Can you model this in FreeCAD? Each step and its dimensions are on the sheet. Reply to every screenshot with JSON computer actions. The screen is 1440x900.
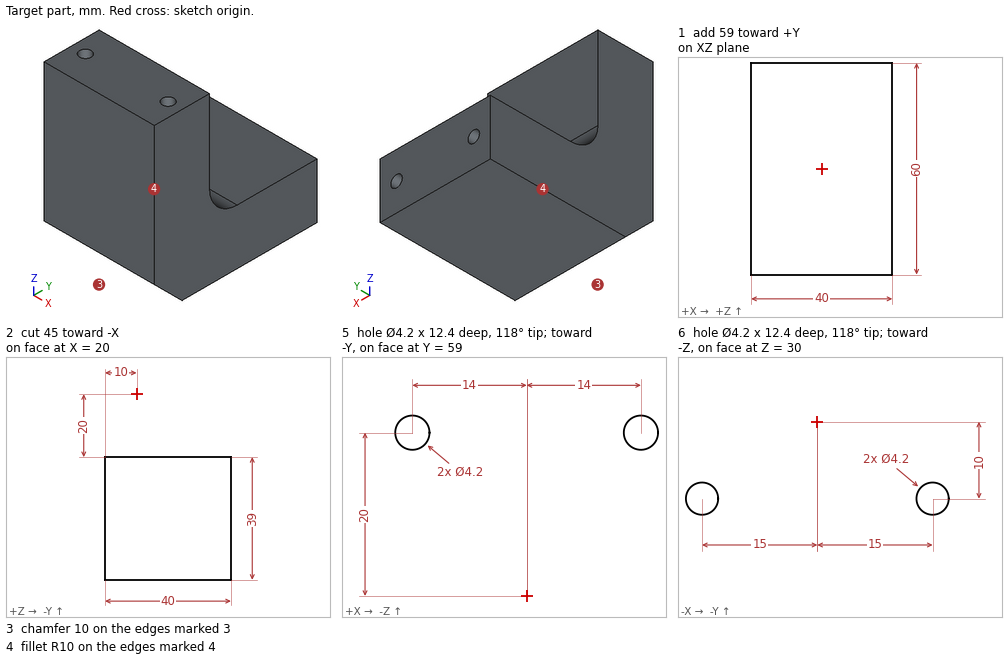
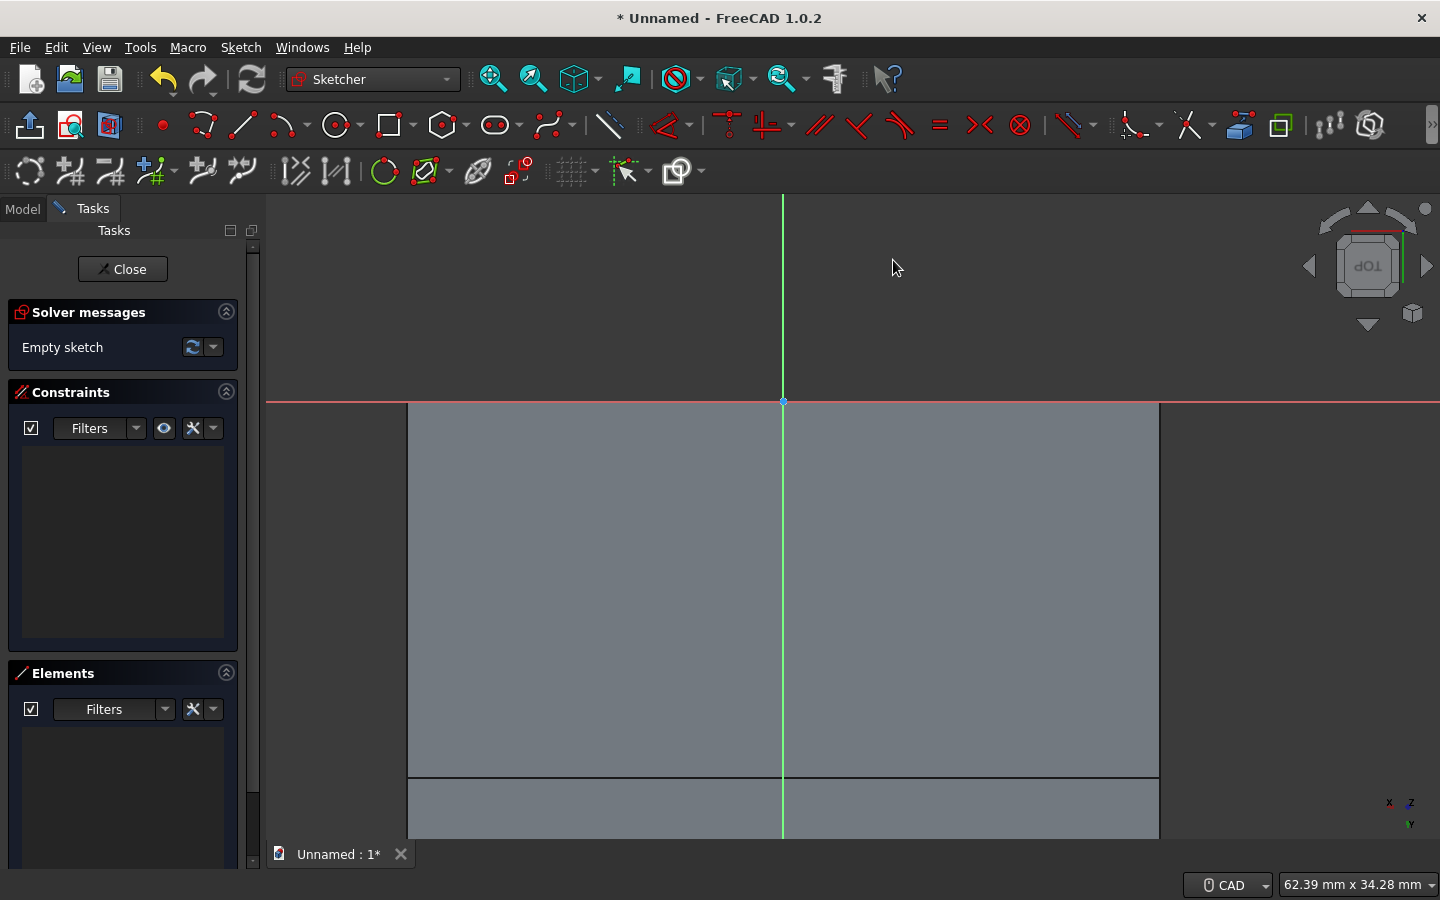
{"action": "left_click", "coordinate": [336, 126]}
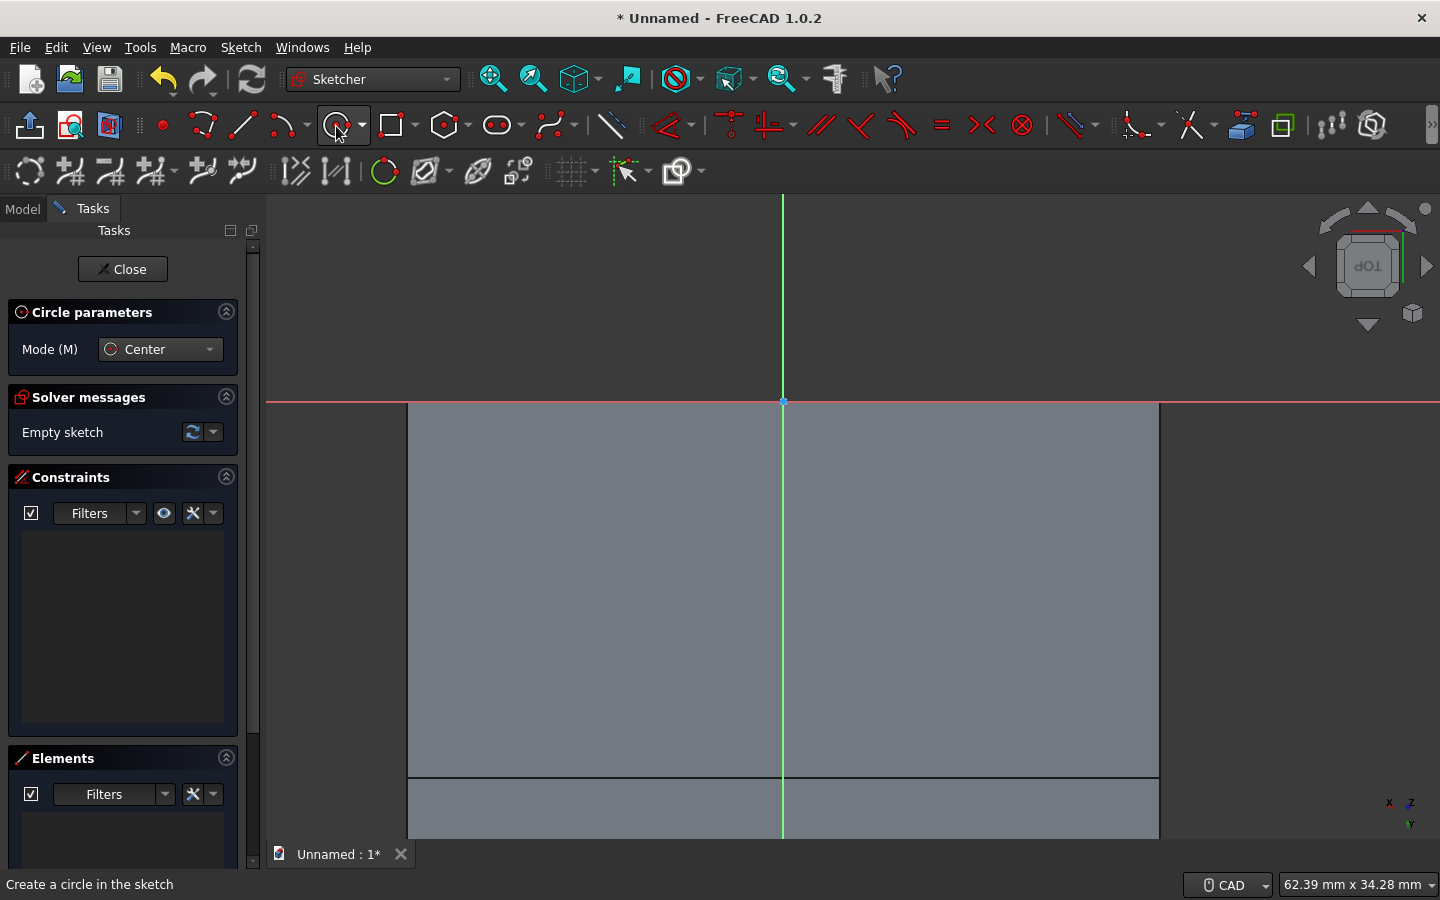
{"action": "left_click", "coordinate": [1066, 590]}
{"action": "mouse_move", "coordinate": [1094, 562]}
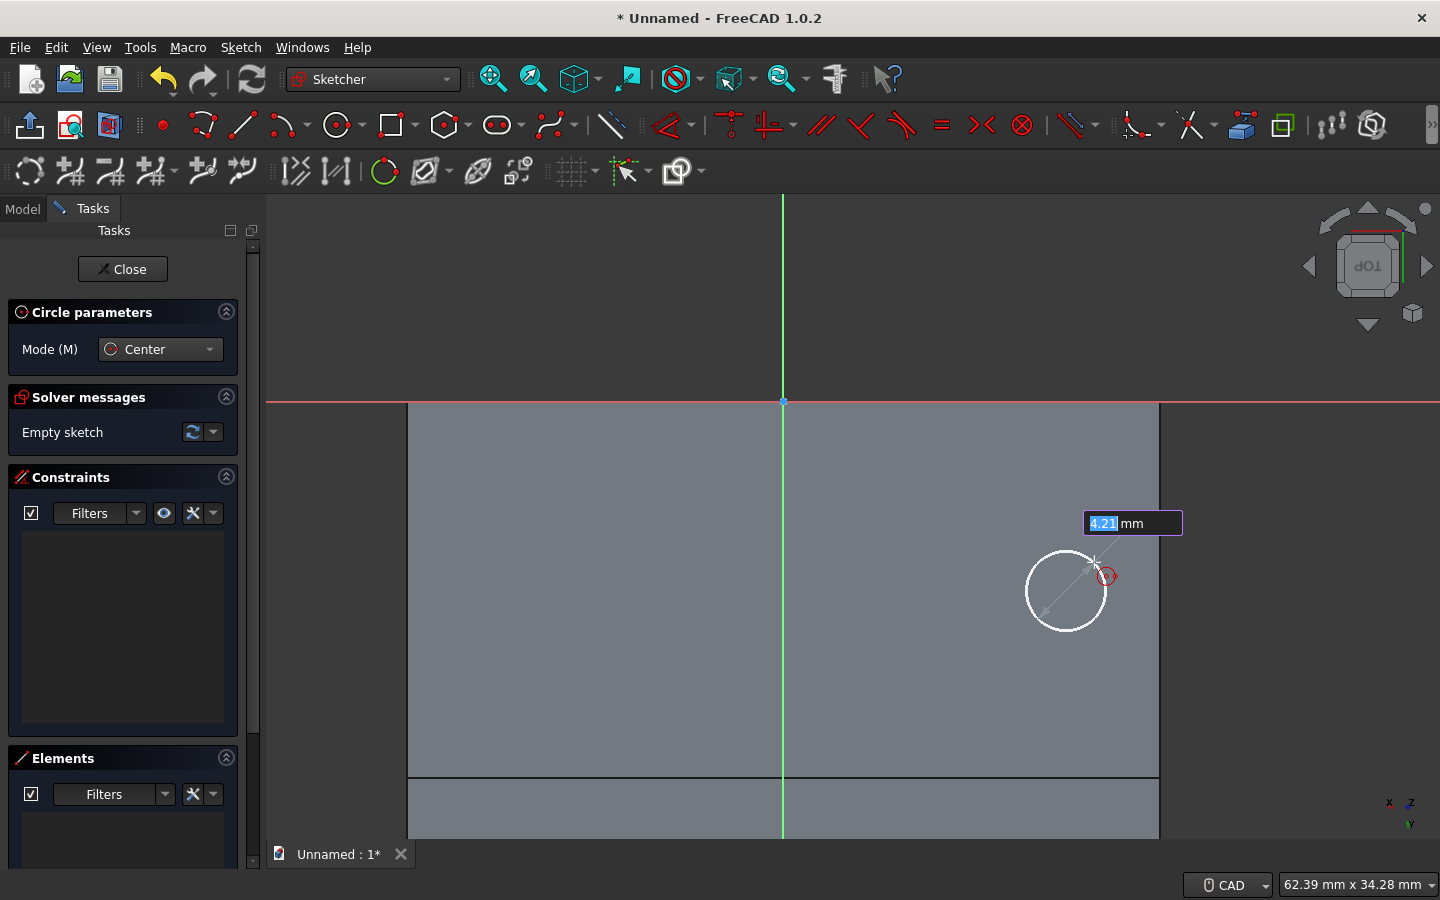
{"action": "type", "text": "4.2"}
{"action": "key", "text": "Return"}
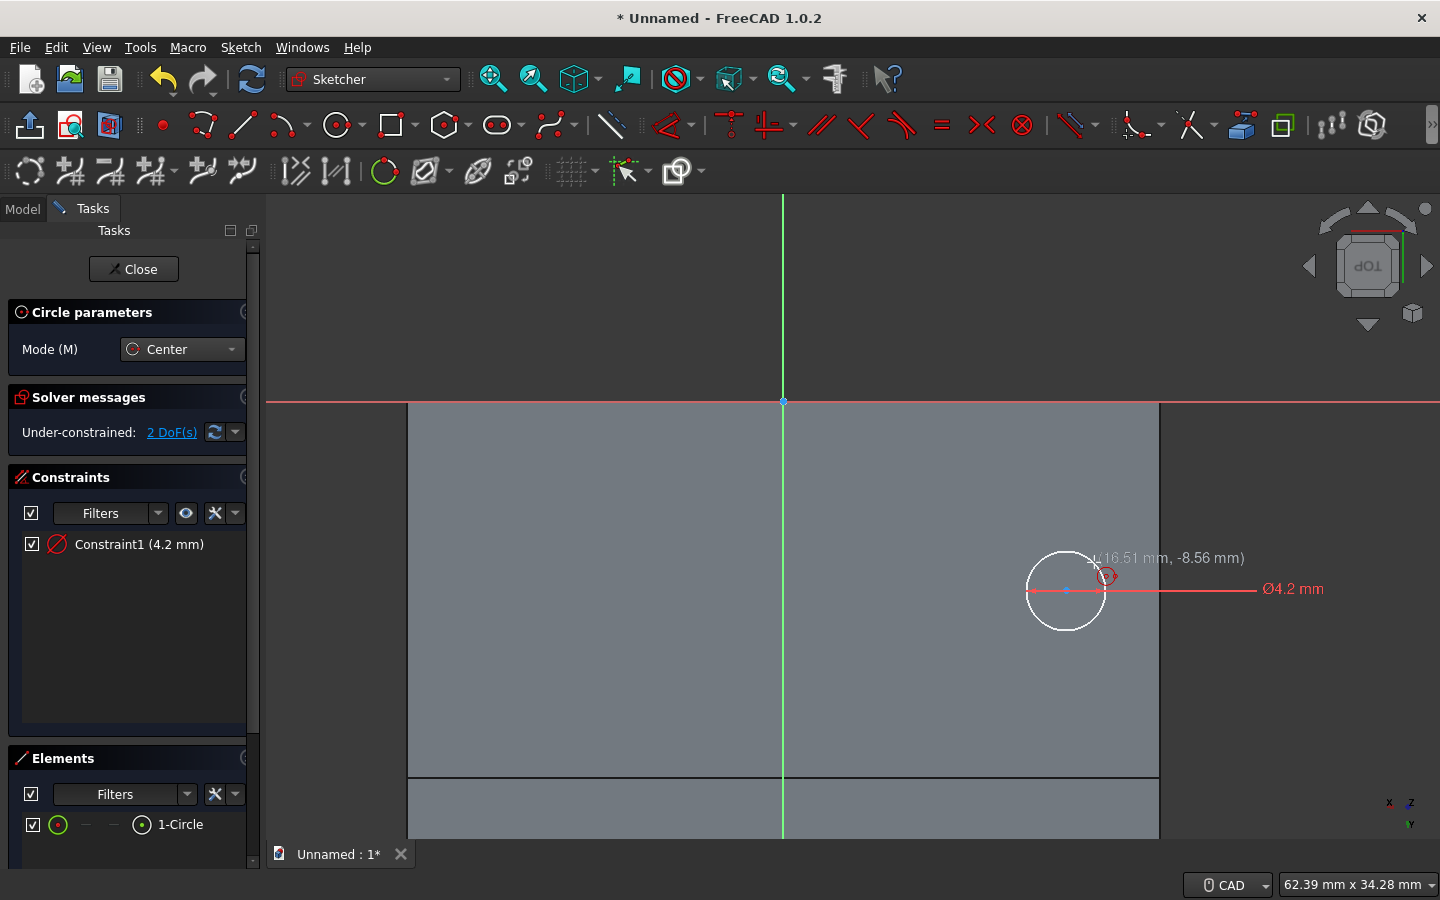
{"action": "left_click", "coordinate": [501, 590]}
{"action": "mouse_move", "coordinate": [529, 562]}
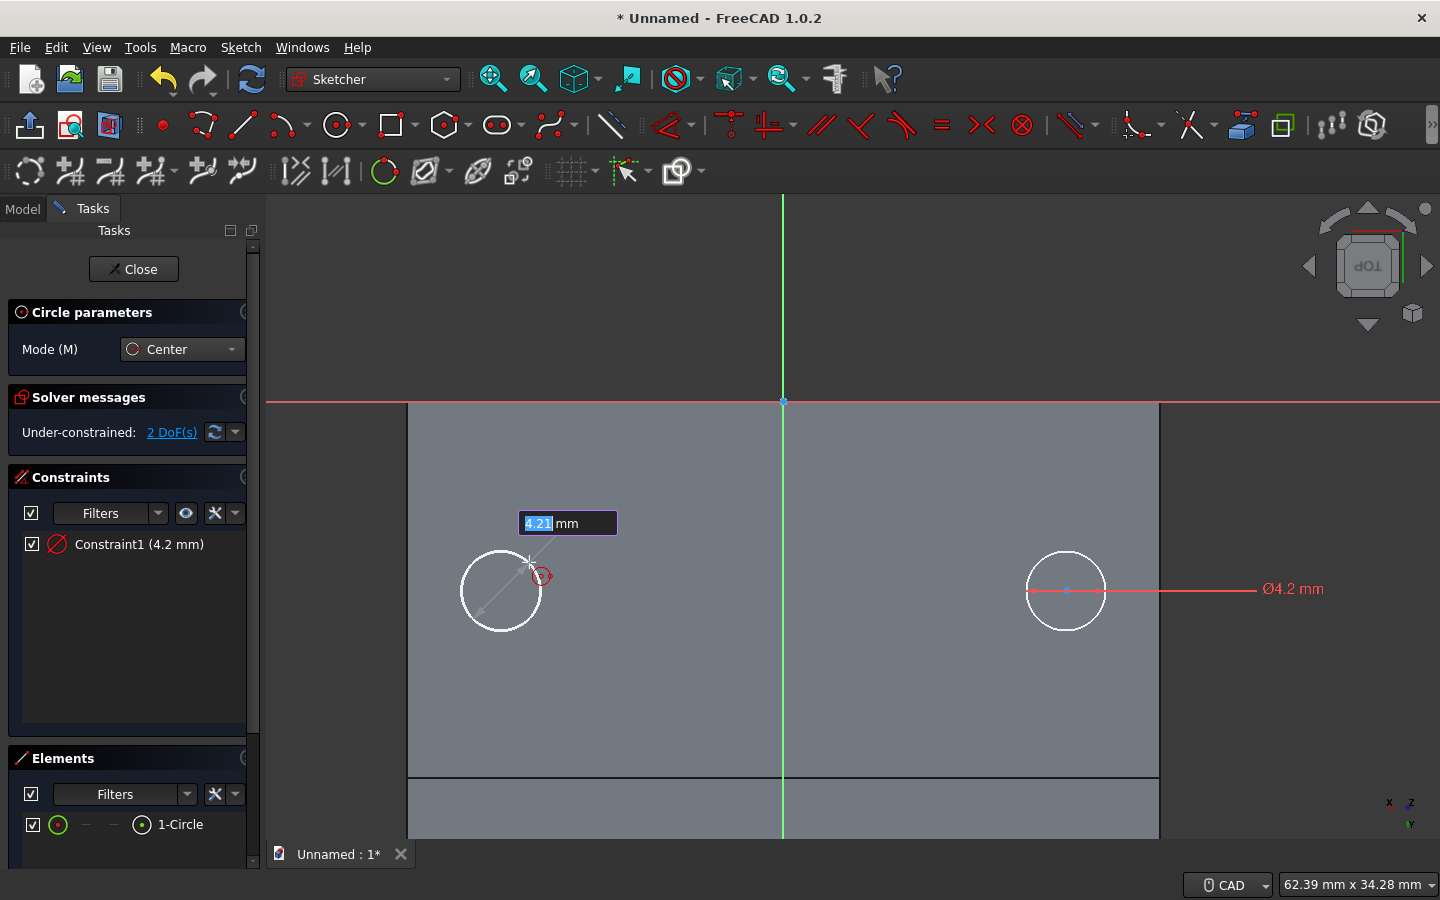
{"action": "type", "text": "4.2"}
{"action": "key", "text": "Return"}
{"action": "key", "text": "Escape"}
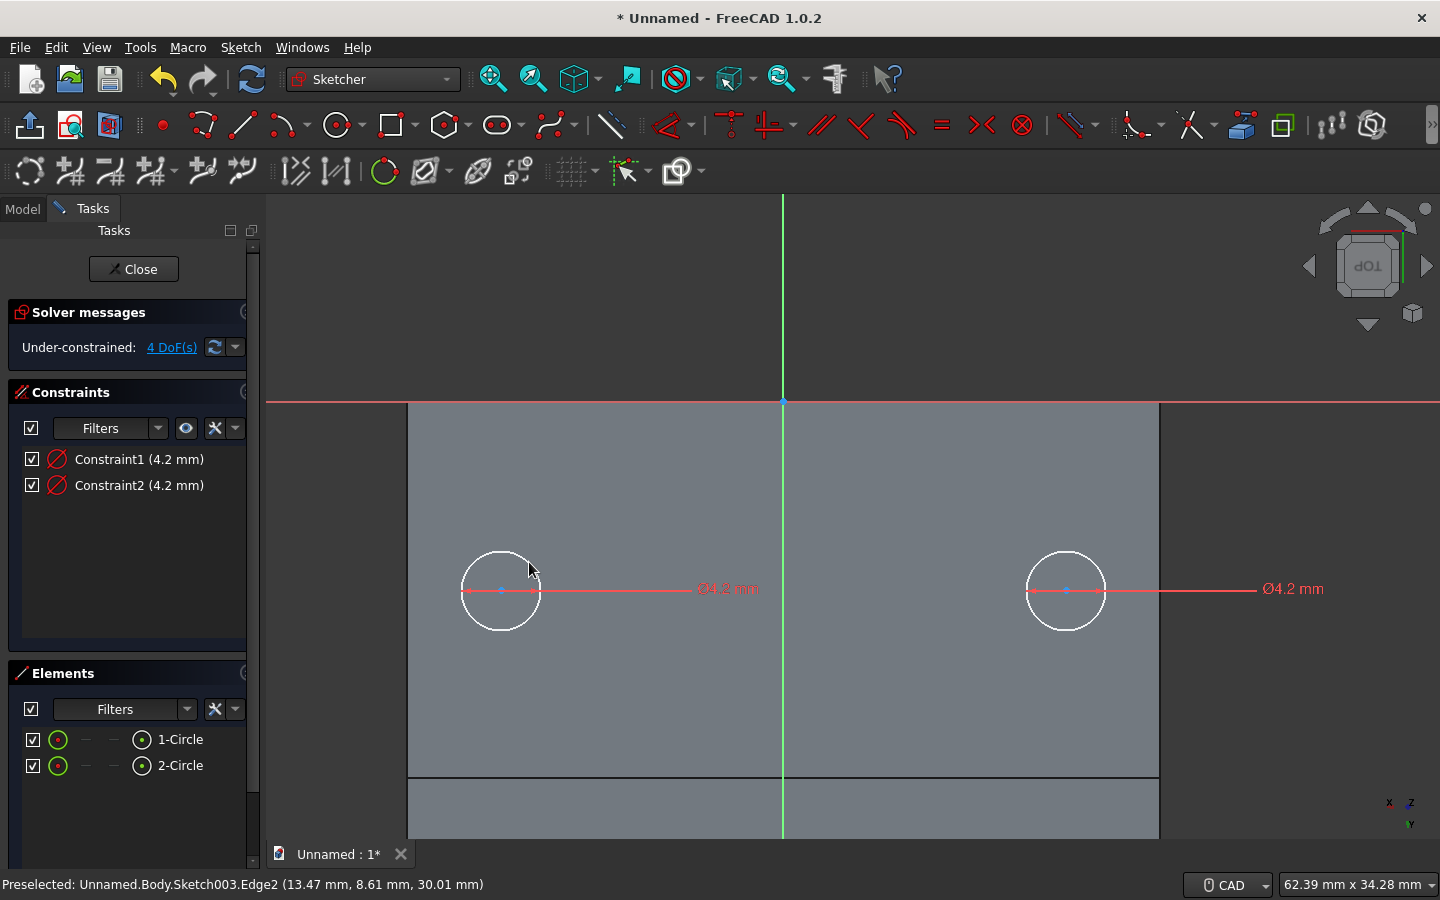
{"action": "left_click", "coordinate": [1066, 591]}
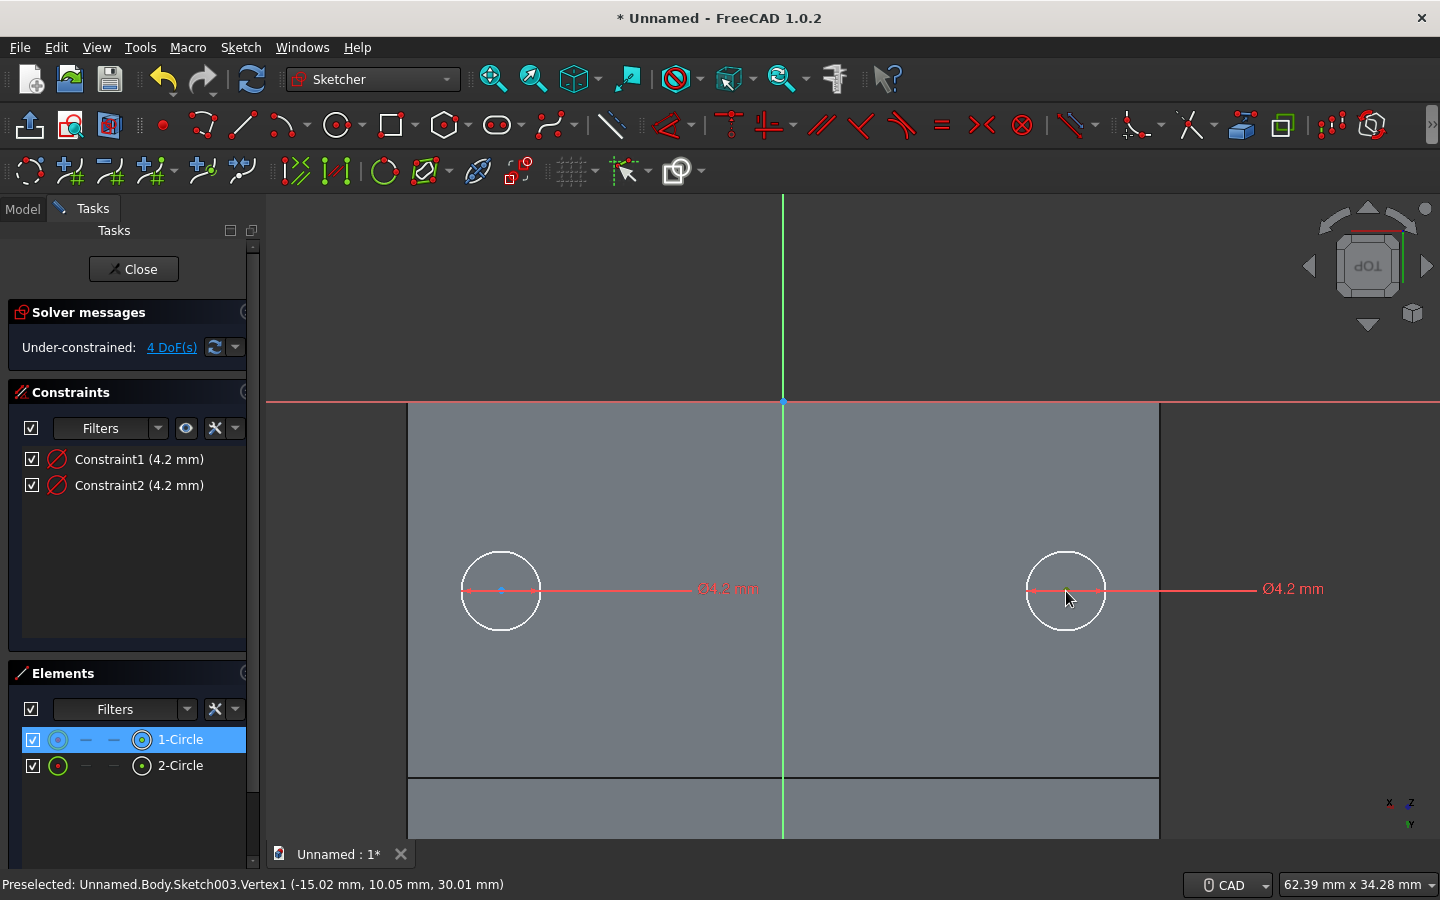
{"action": "left_click", "coordinate": [501, 591]}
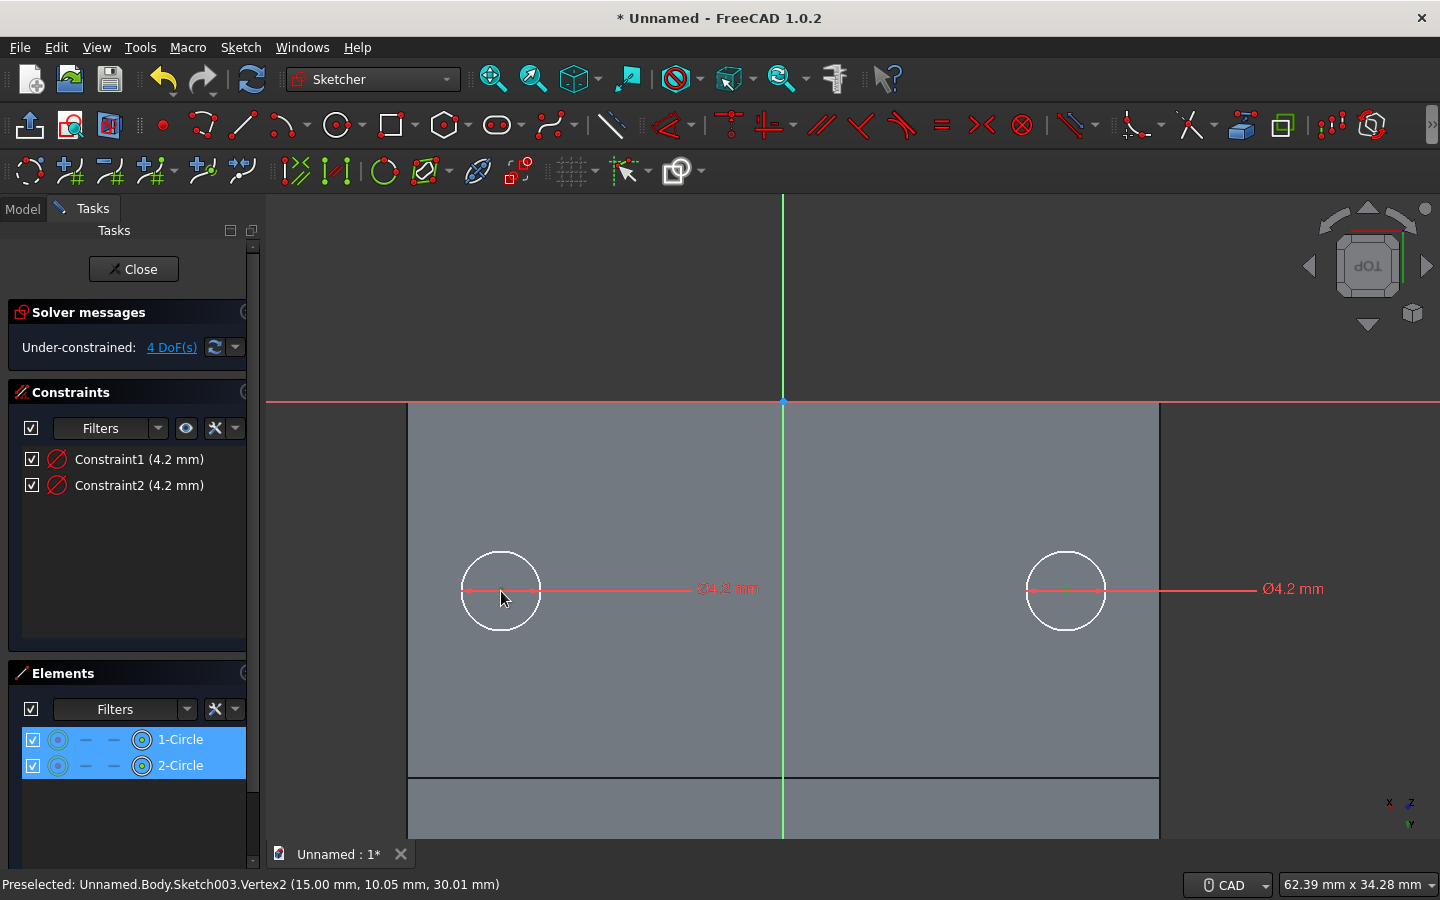
{"action": "key", "text": "h"}